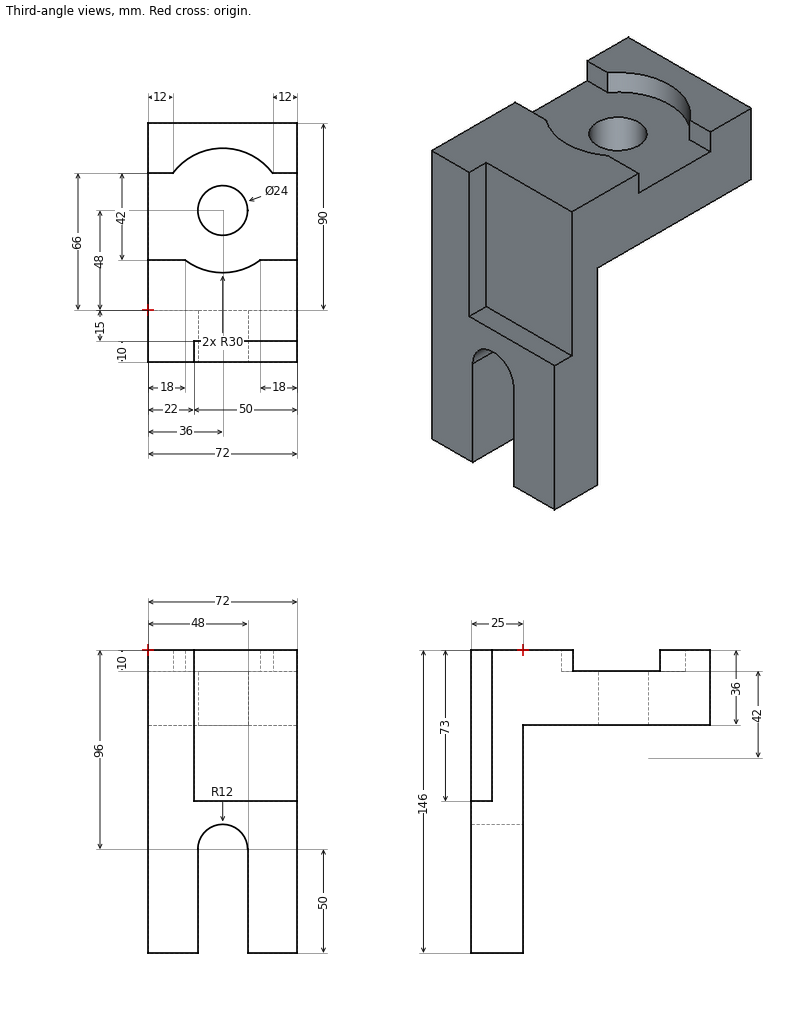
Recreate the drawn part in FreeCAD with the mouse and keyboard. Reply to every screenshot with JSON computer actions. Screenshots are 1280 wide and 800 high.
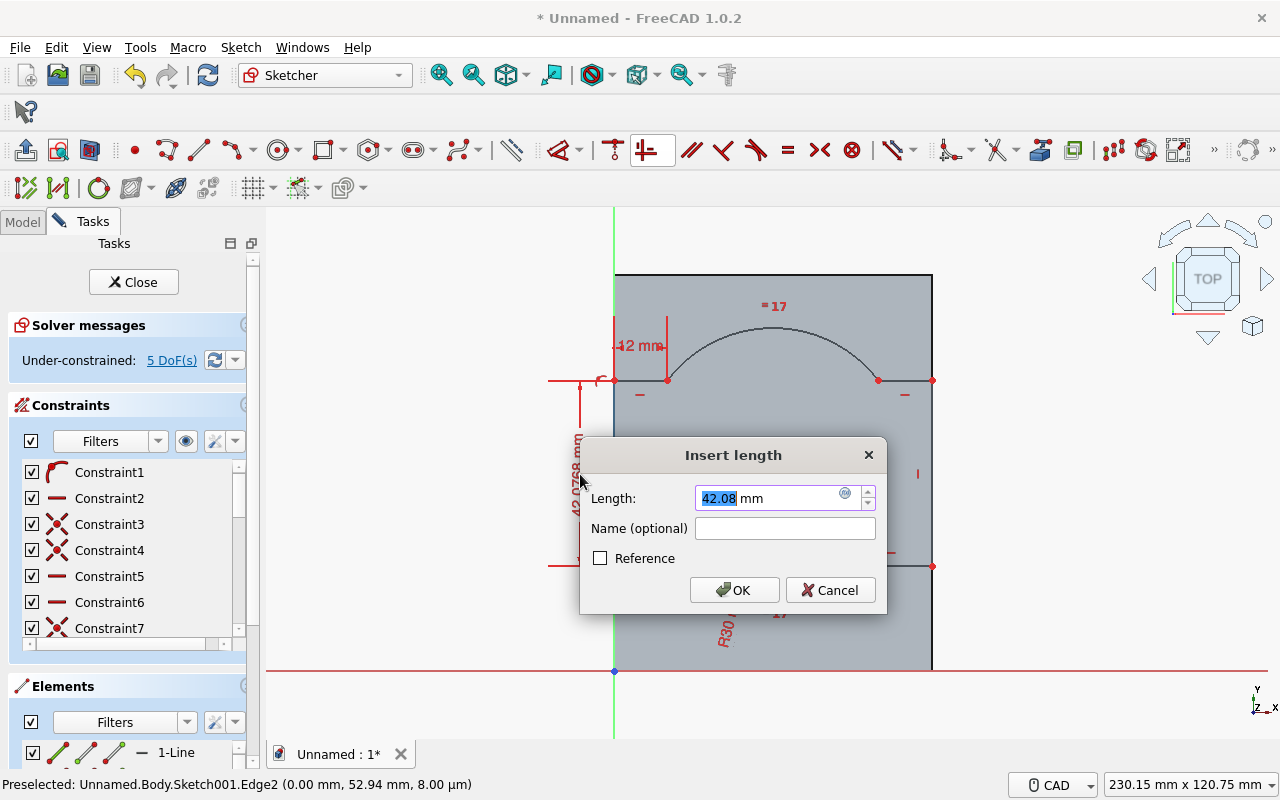
{"action": "type", "text": "42"}
{"action": "key", "text": "Return"}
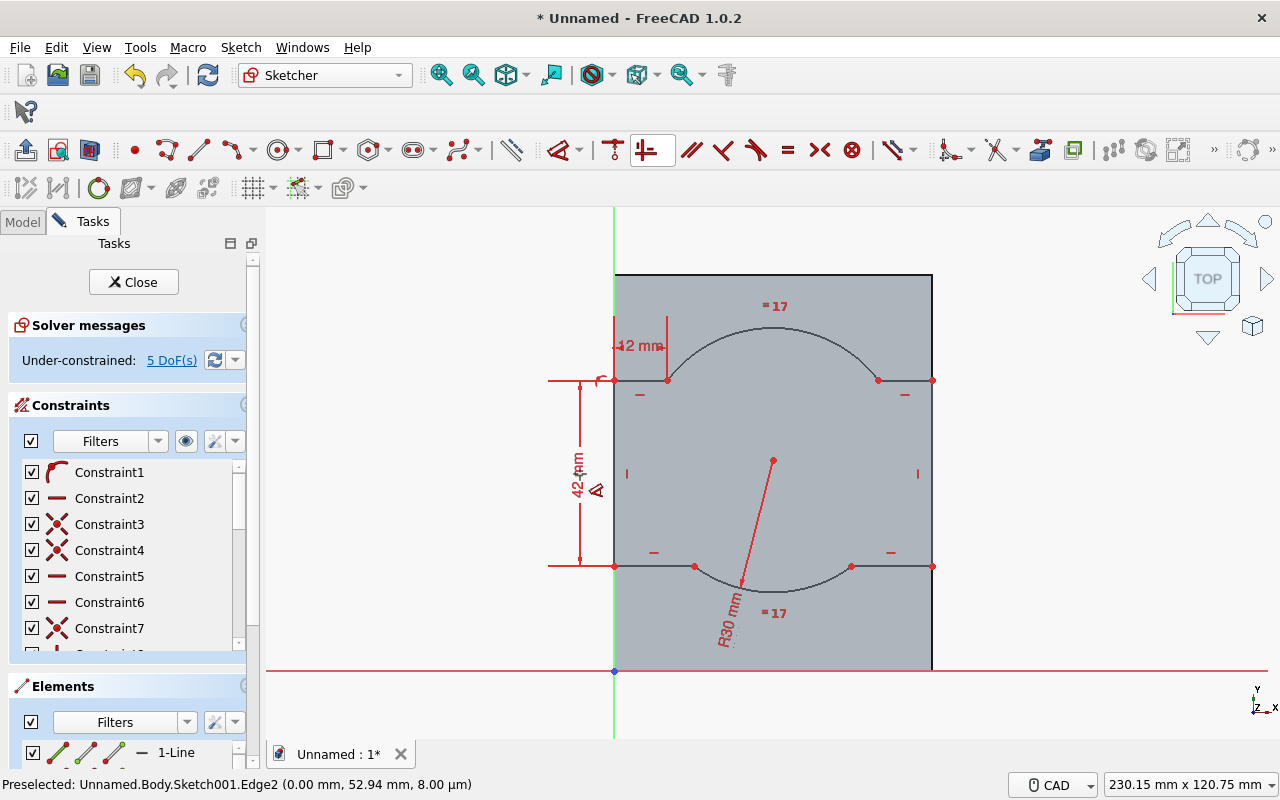
{"action": "left_click", "coordinate": [638, 566]}
{"action": "left_click", "coordinate": [654, 600]}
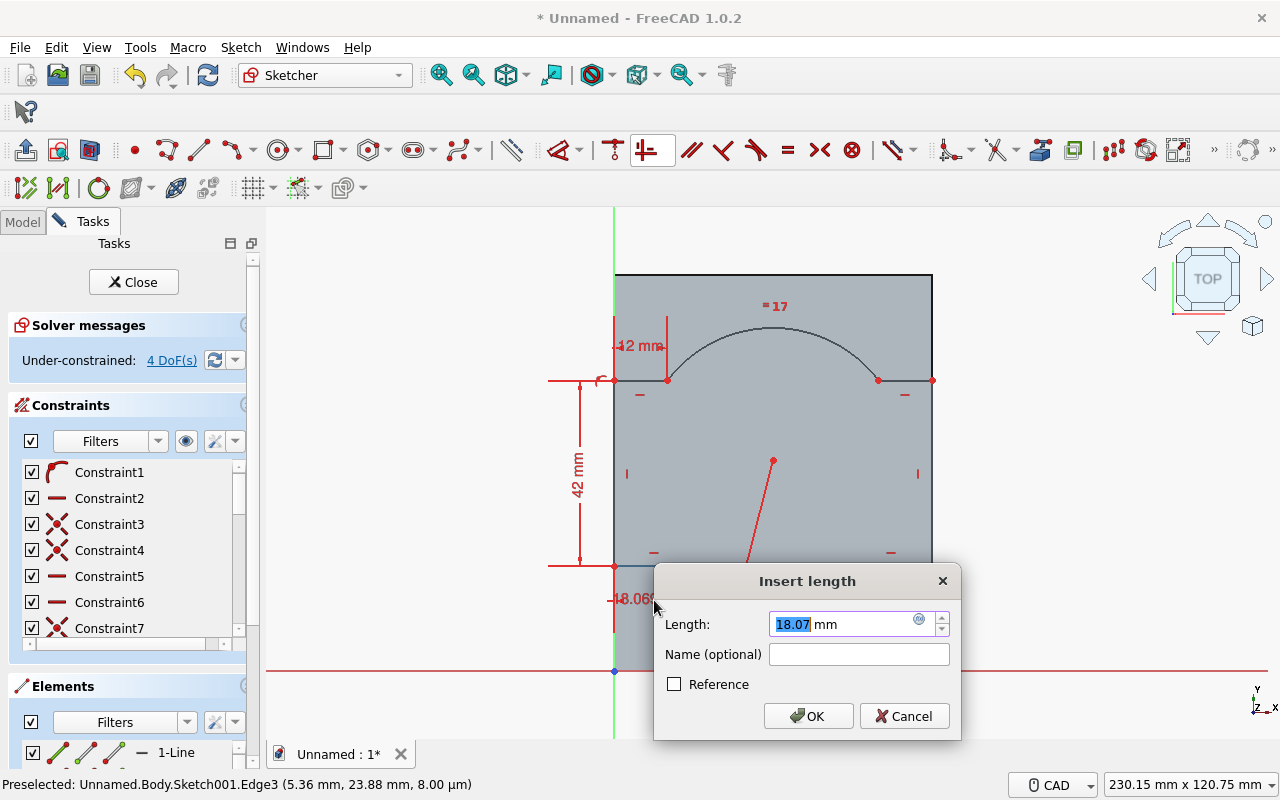
{"action": "type", "text": "18"}
{"action": "key", "text": "Return"}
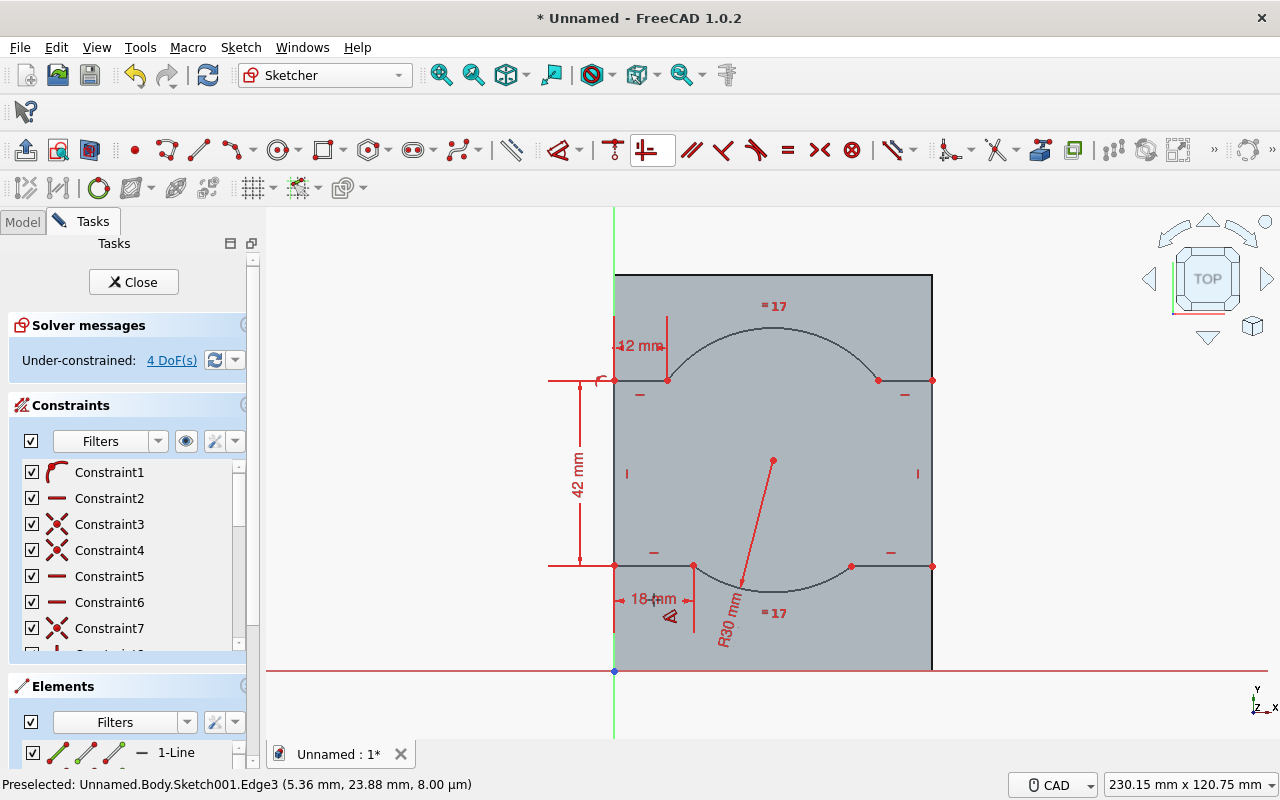
{"action": "left_click", "coordinate": [876, 566]}
{"action": "left_click", "coordinate": [892, 600]}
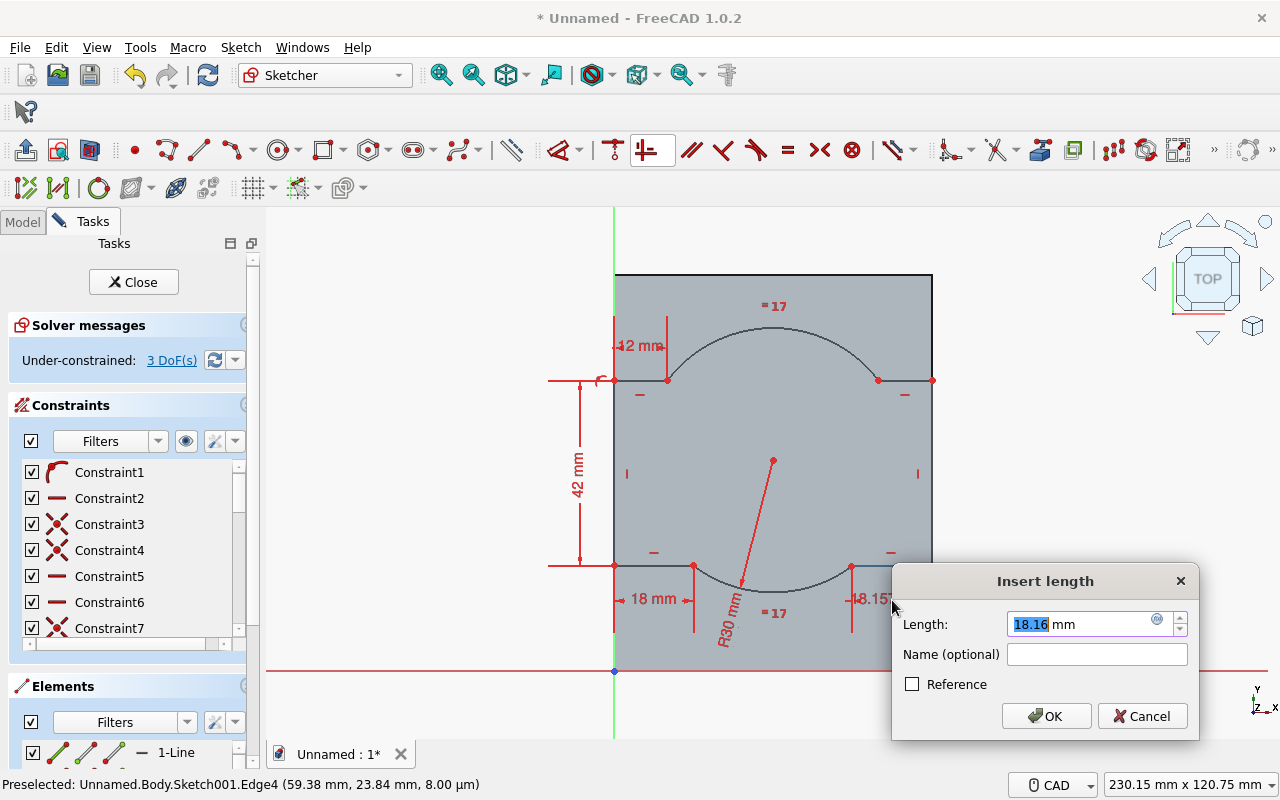
{"action": "type", "text": "18"}
{"action": "key", "text": "Return"}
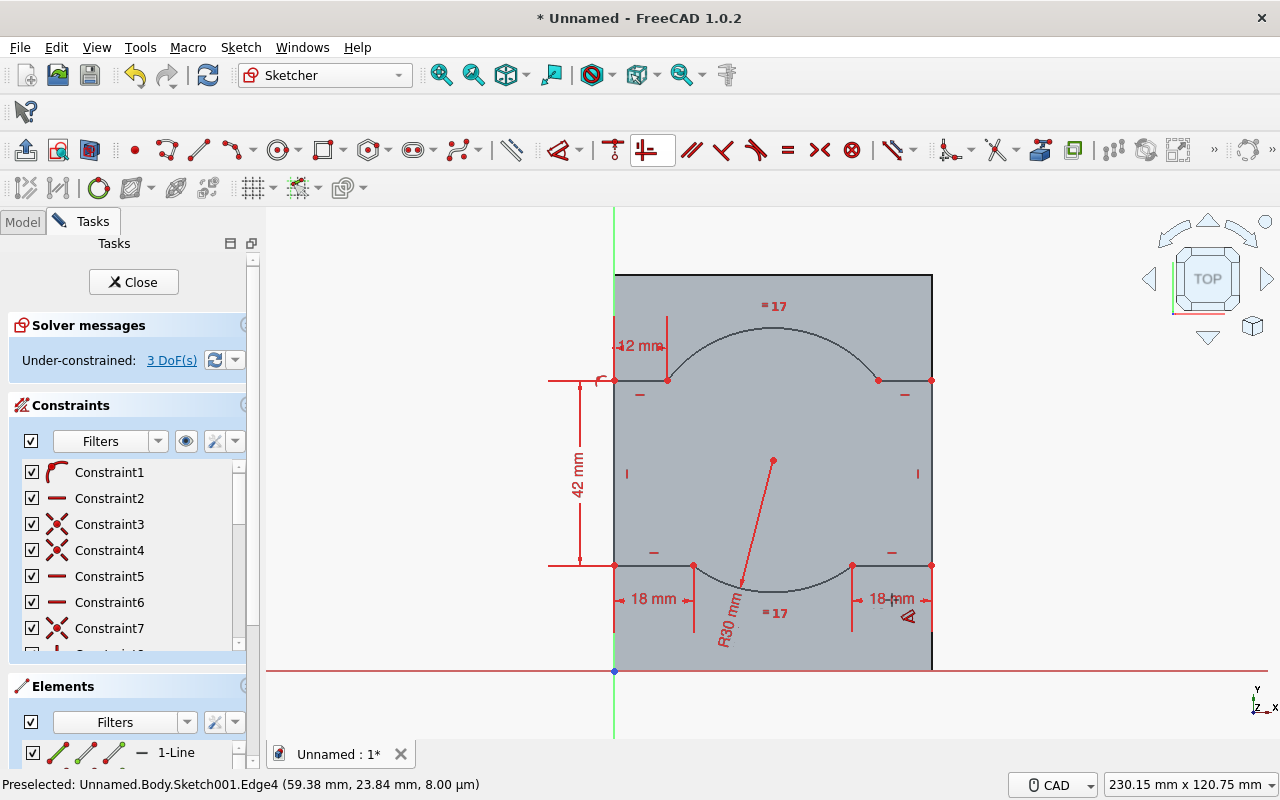
{"action": "left_click", "coordinate": [932, 510]}
{"action": "left_click", "coordinate": [966, 473]}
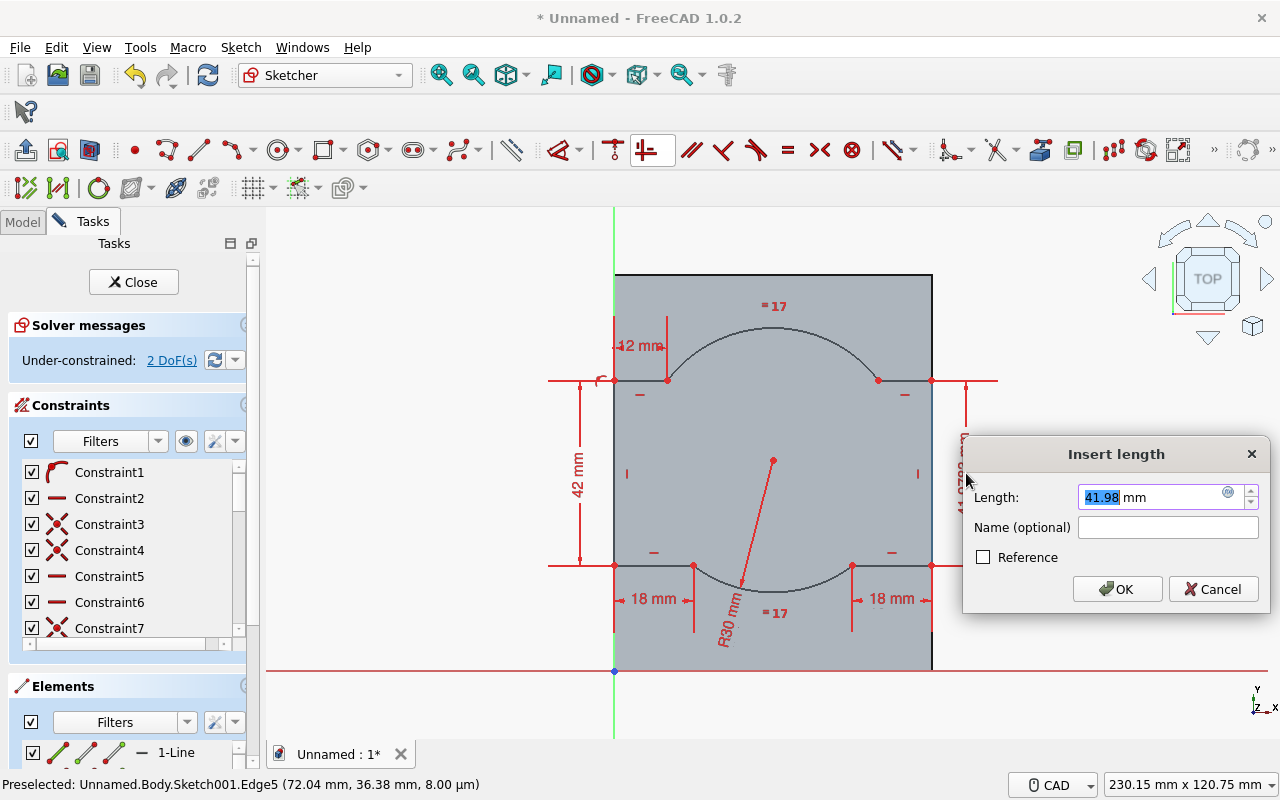
{"action": "type", "text": "42"}
{"action": "key", "text": "Return"}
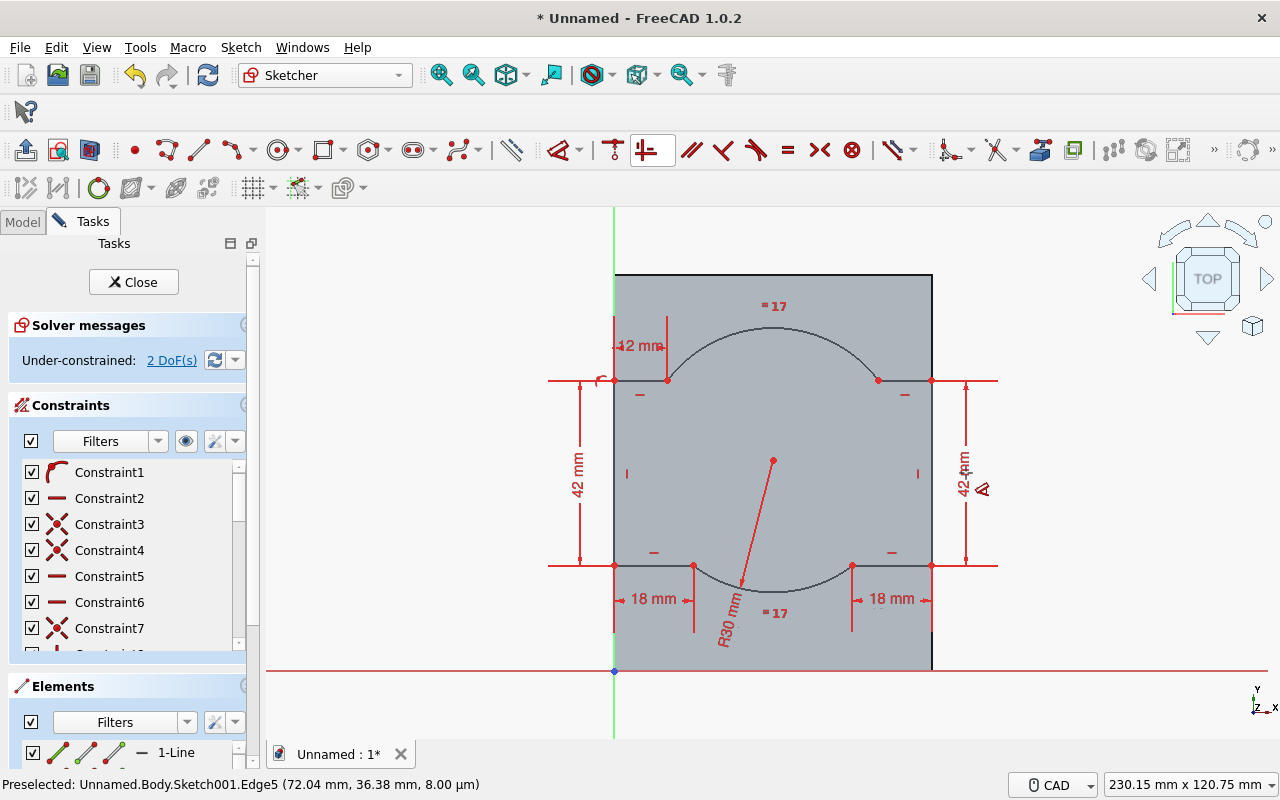
{"action": "left_click", "coordinate": [916, 381]}
{"action": "left_click", "coordinate": [905, 347]}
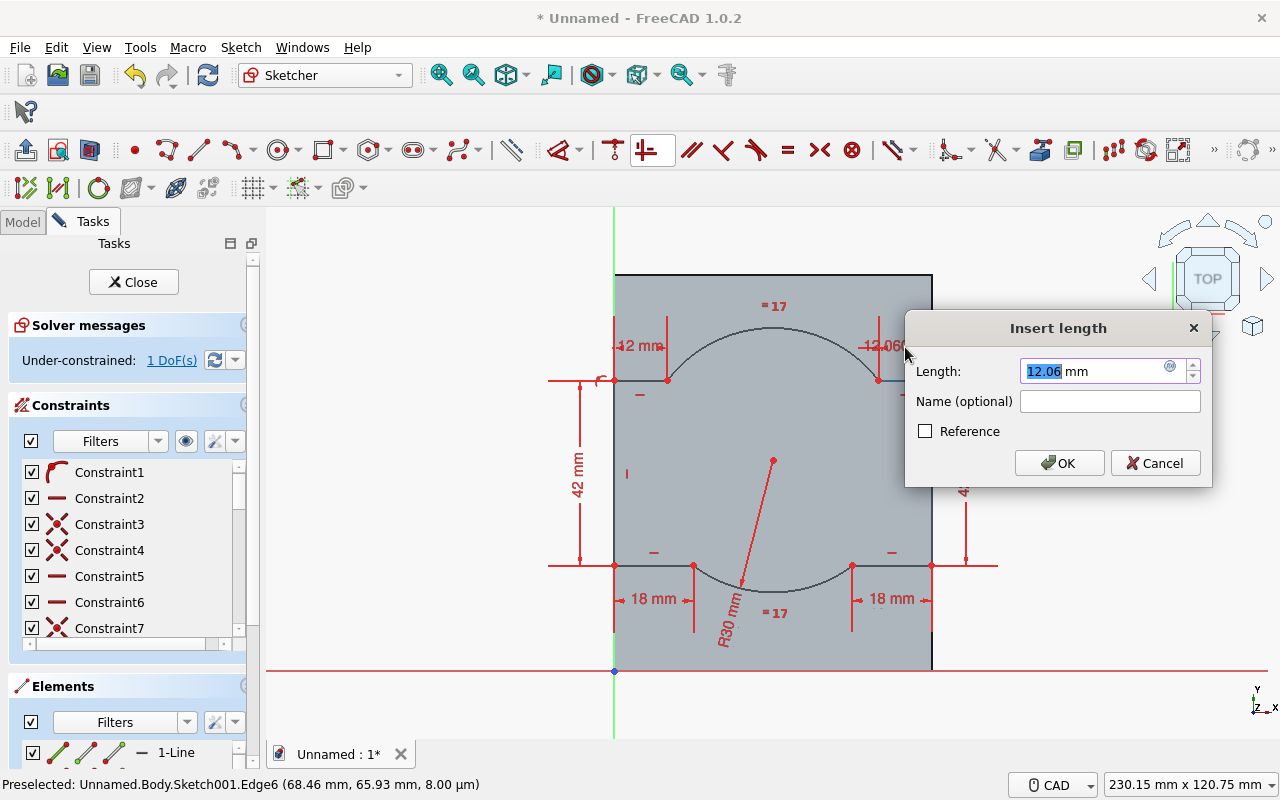
{"action": "type", "text": "12"}
{"action": "key", "text": "Return"}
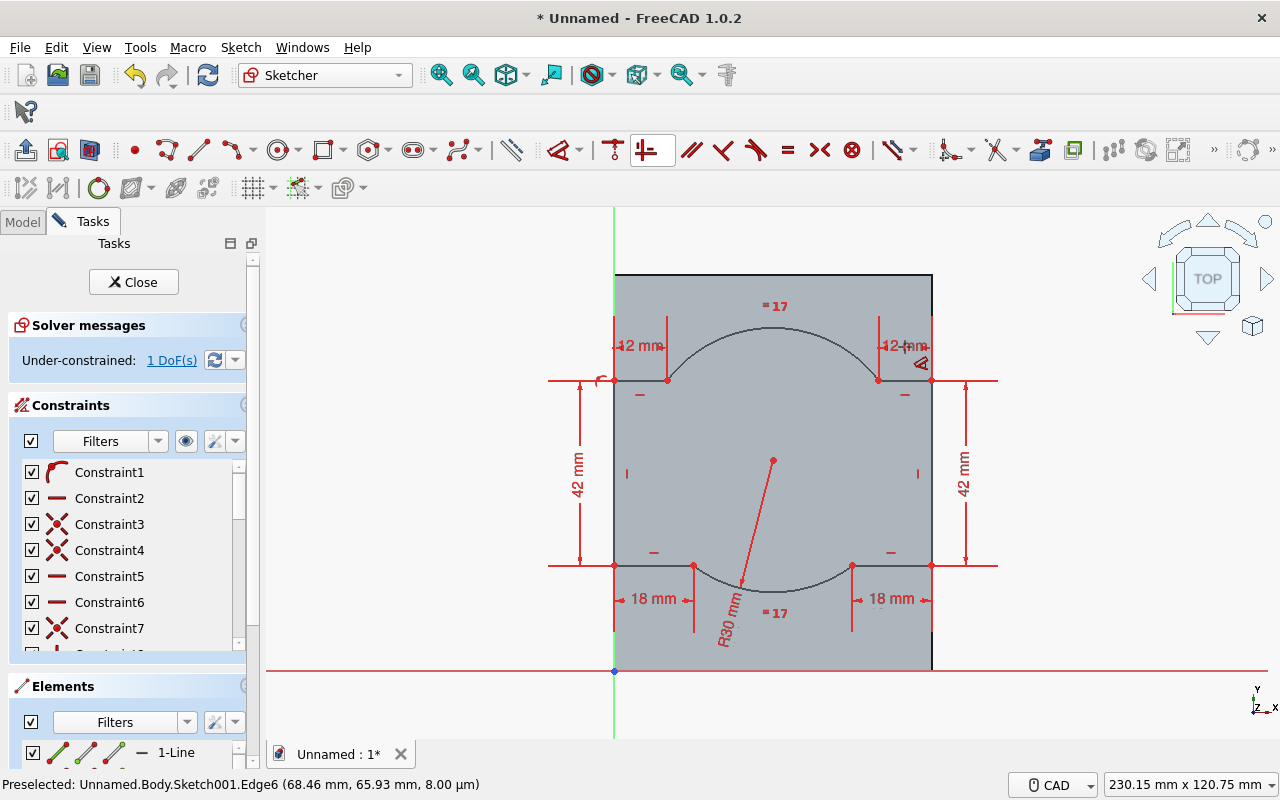
{"action": "left_click", "coordinate": [667, 381]}
{"action": "left_click", "coordinate": [580, 526]}